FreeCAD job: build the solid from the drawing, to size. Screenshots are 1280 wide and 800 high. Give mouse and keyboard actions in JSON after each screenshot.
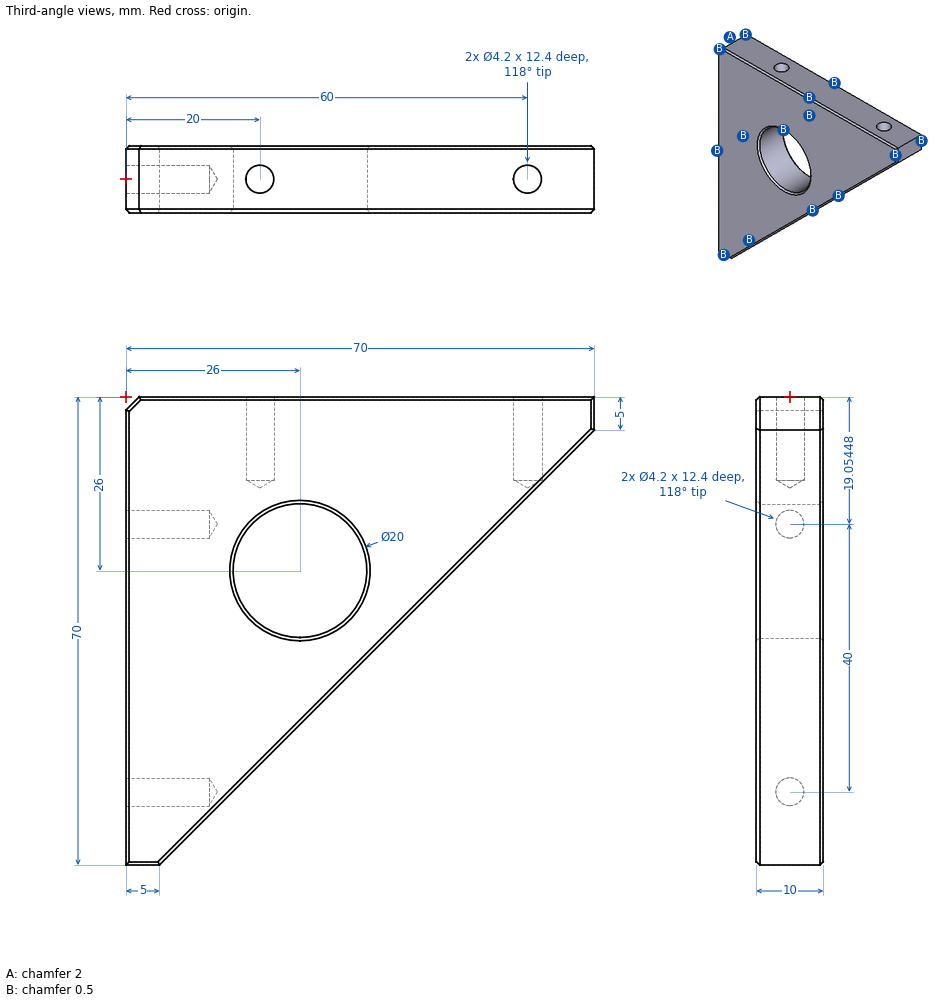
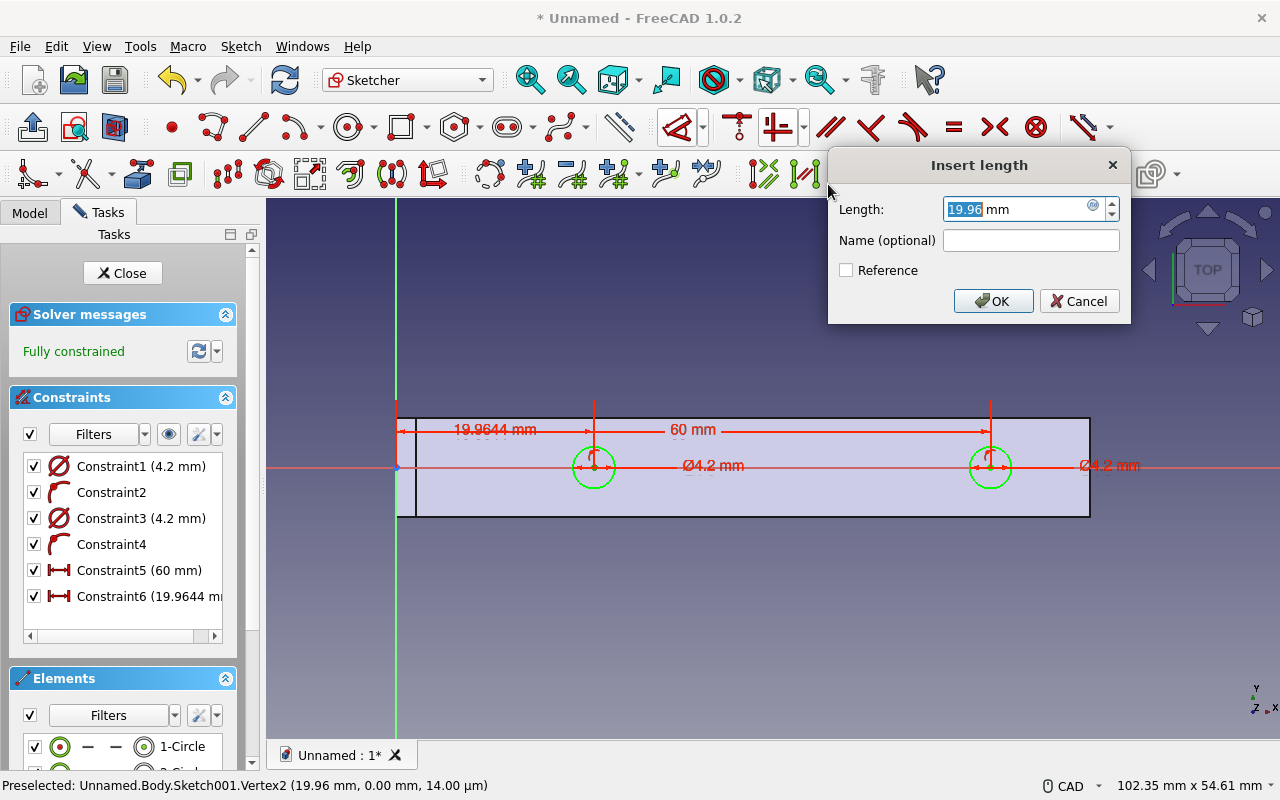
{"action": "type", "text": "20"}
{"action": "key", "text": "Return"}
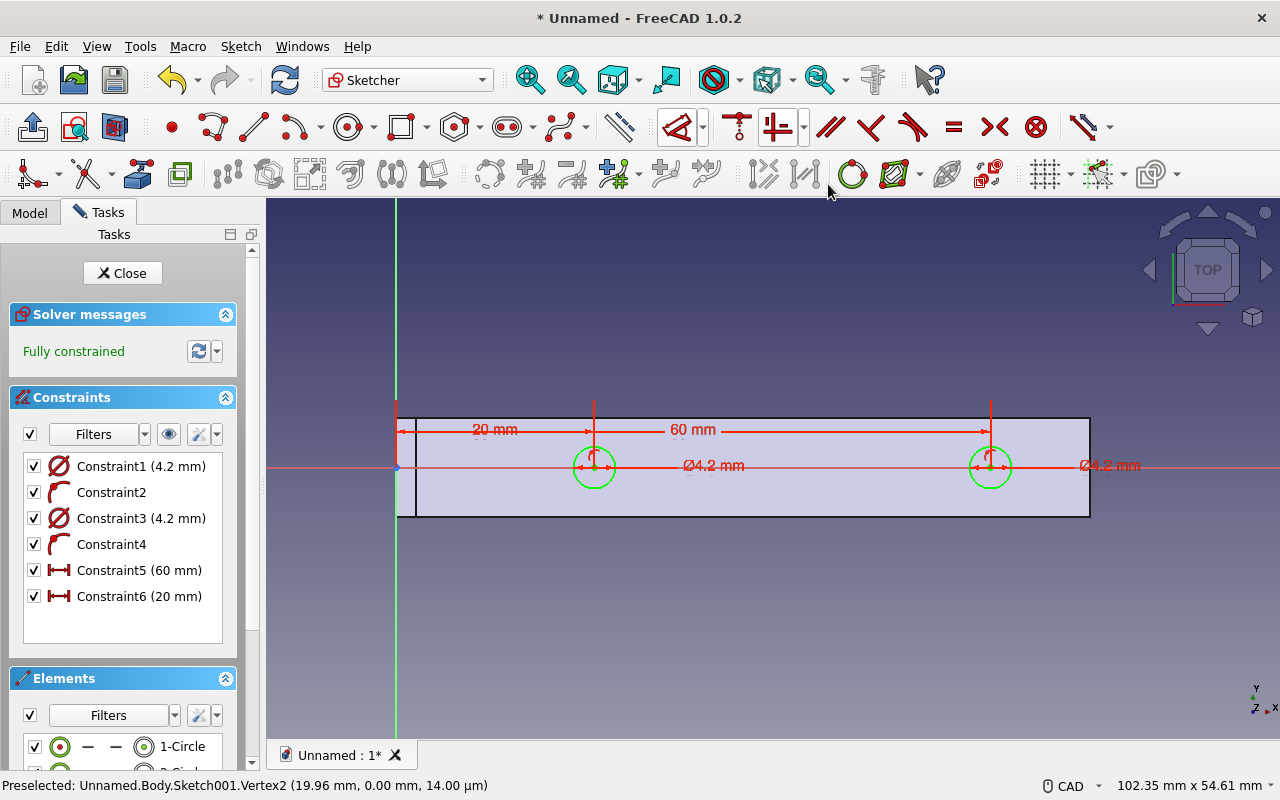
{"action": "left_click", "coordinate": [123, 273]}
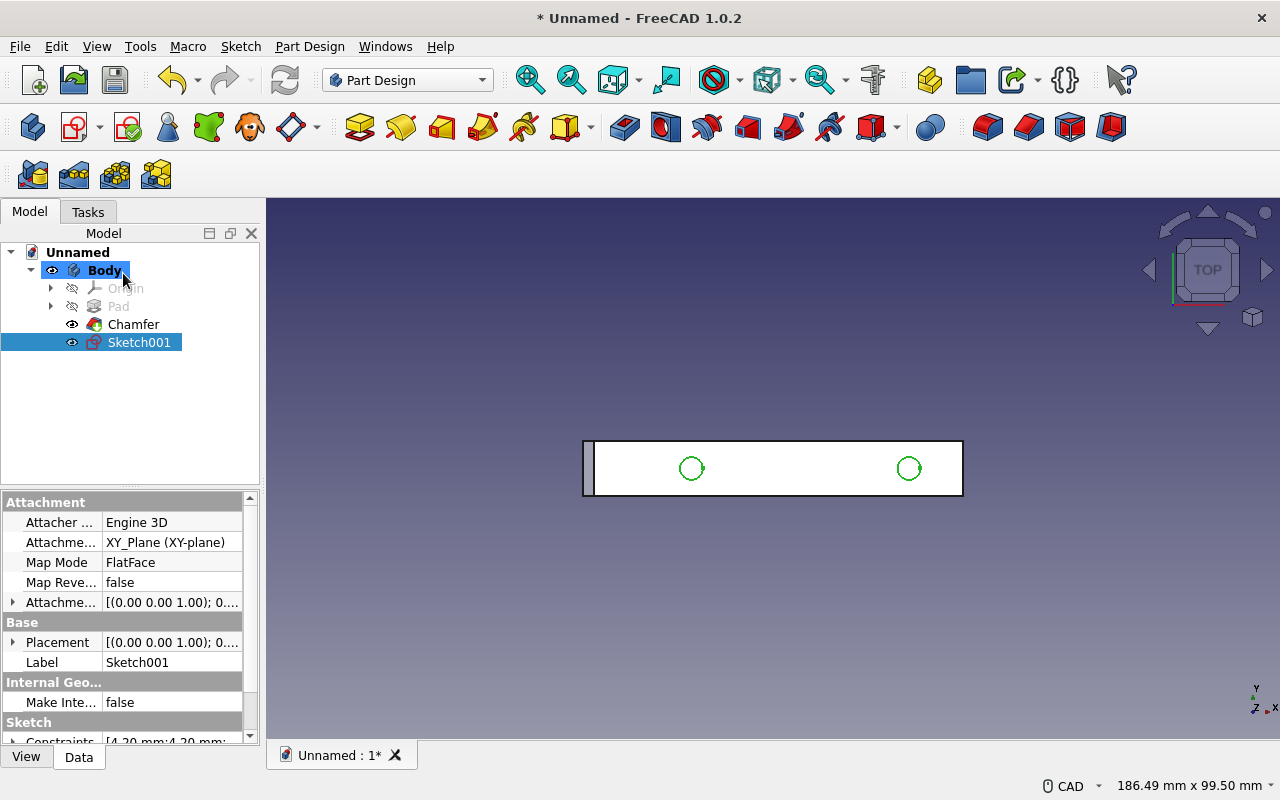
{"action": "left_click", "coordinate": [666, 128]}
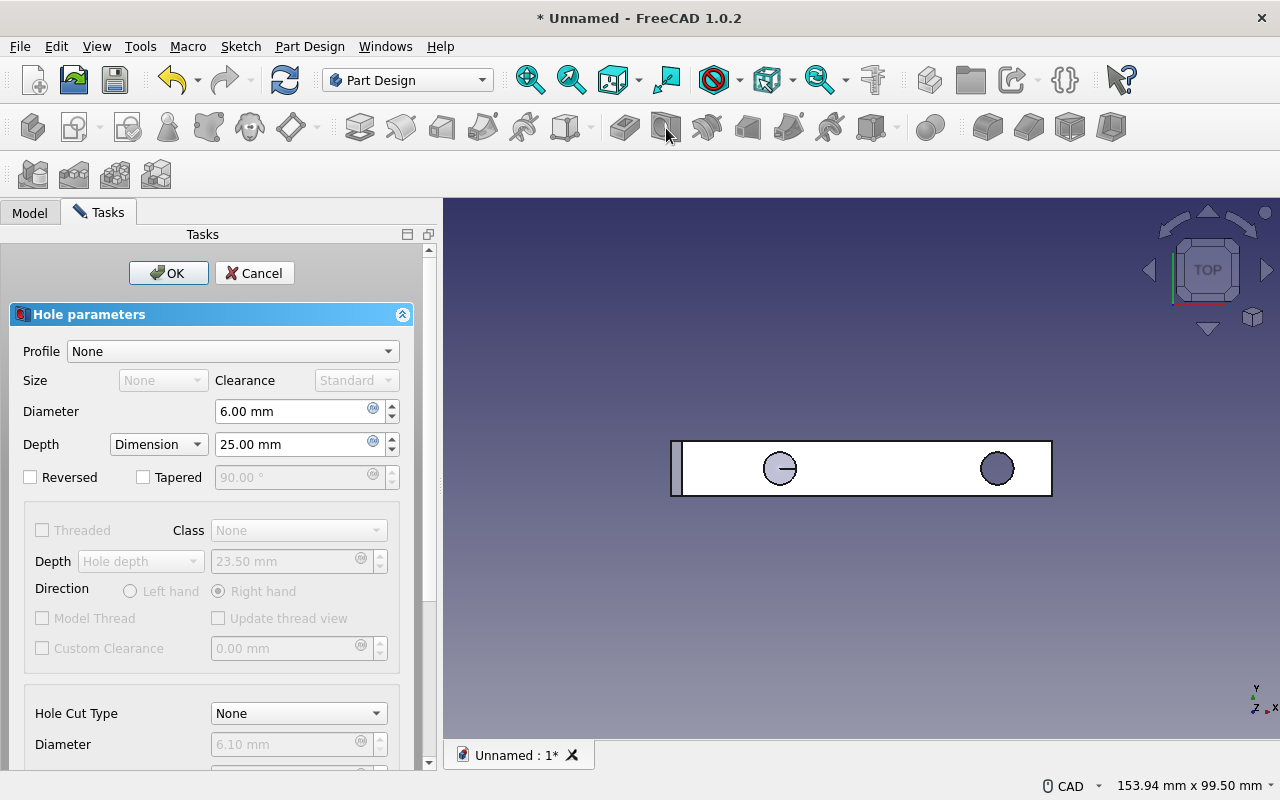
{"action": "triple_click", "coordinate": [300, 412]}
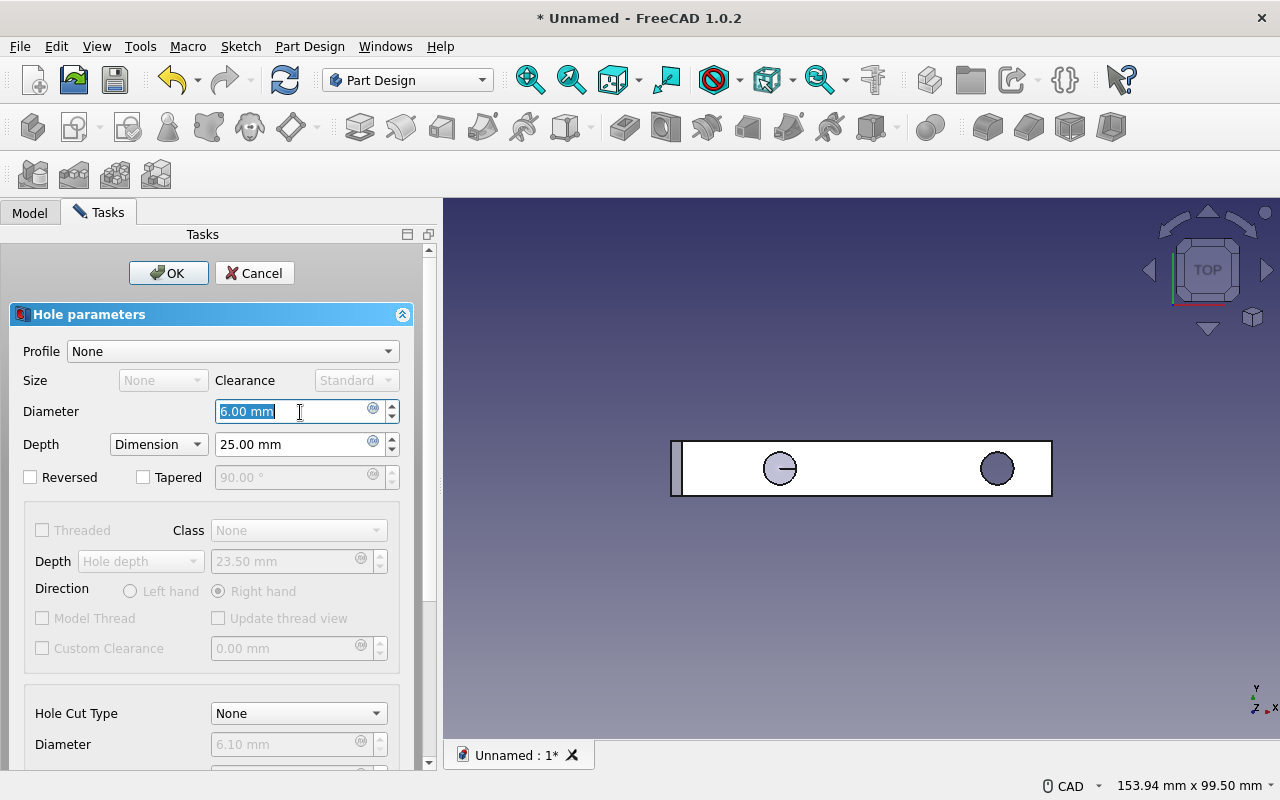
{"action": "type", "text": "4.2"}
{"action": "key", "text": "Tab"}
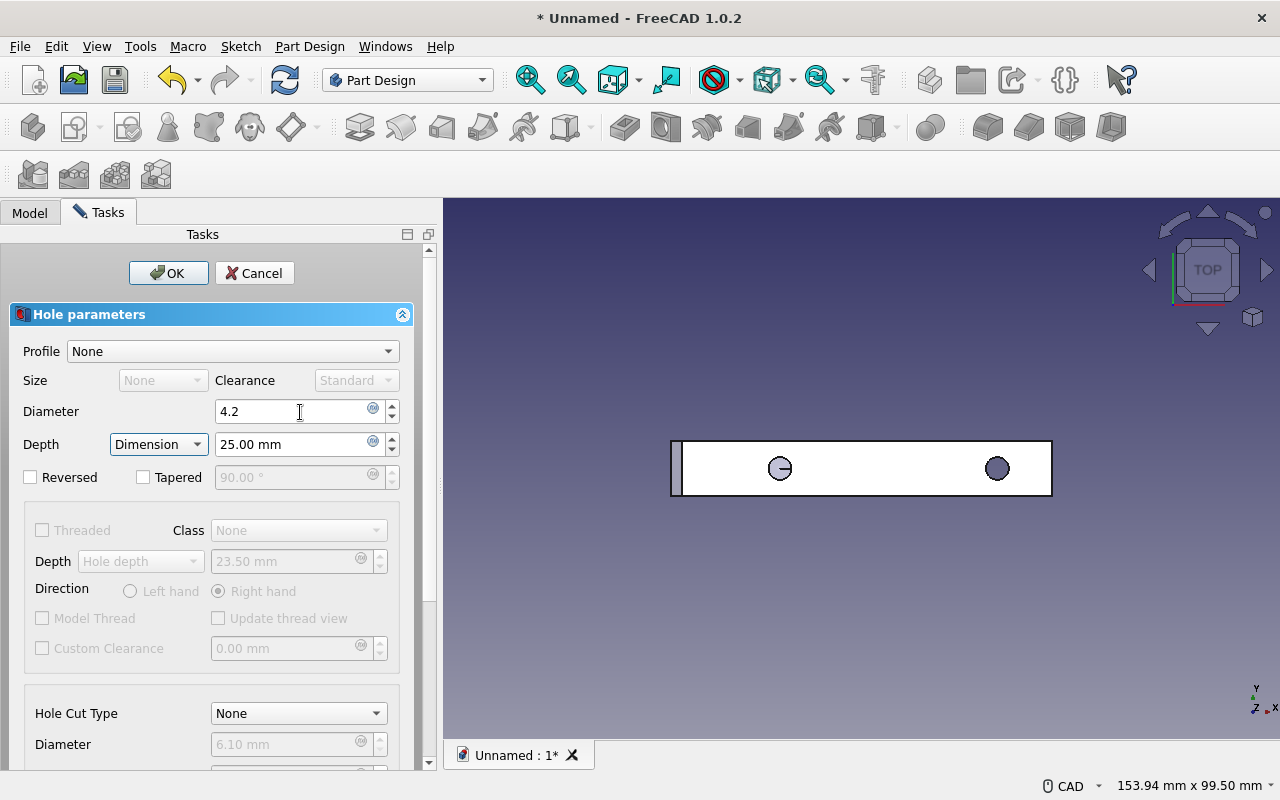
{"action": "triple_click", "coordinate": [300, 444]}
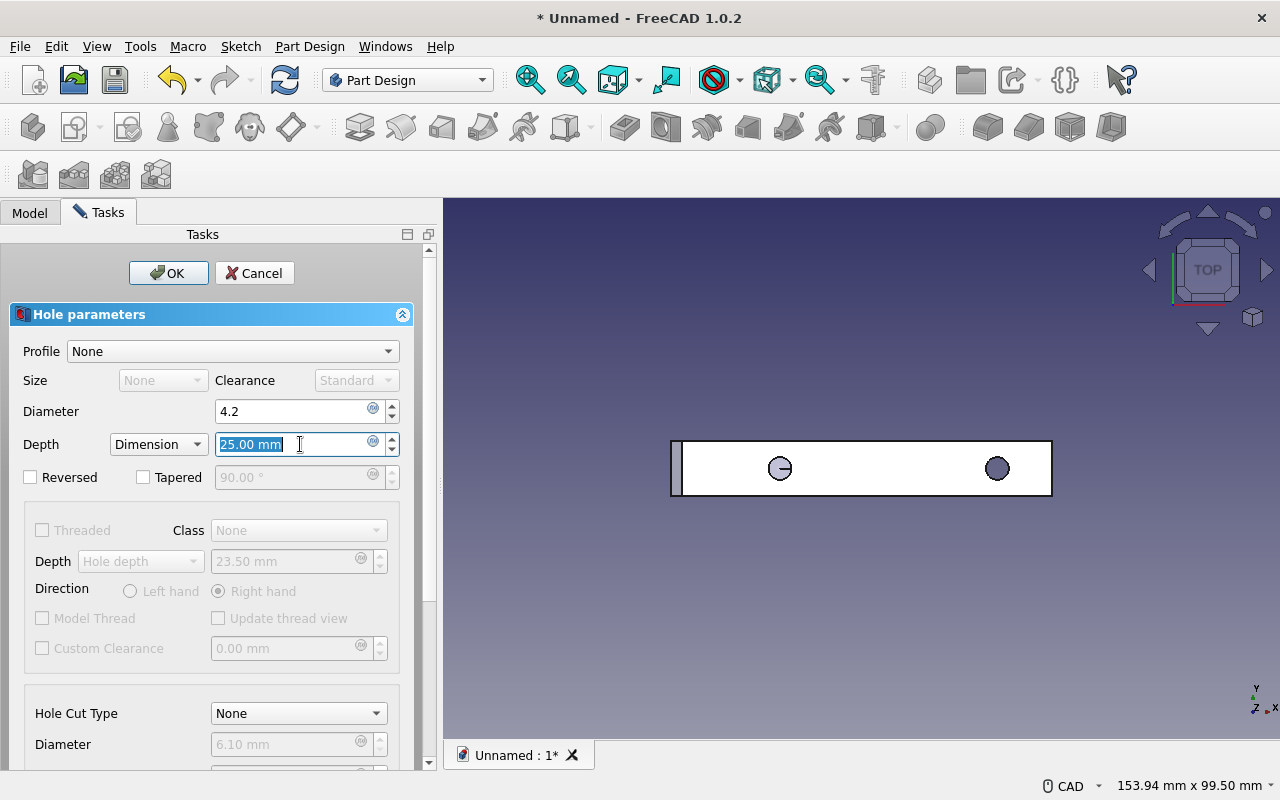
{"action": "type", "text": "12.4"}
{"action": "key", "text": "Tab"}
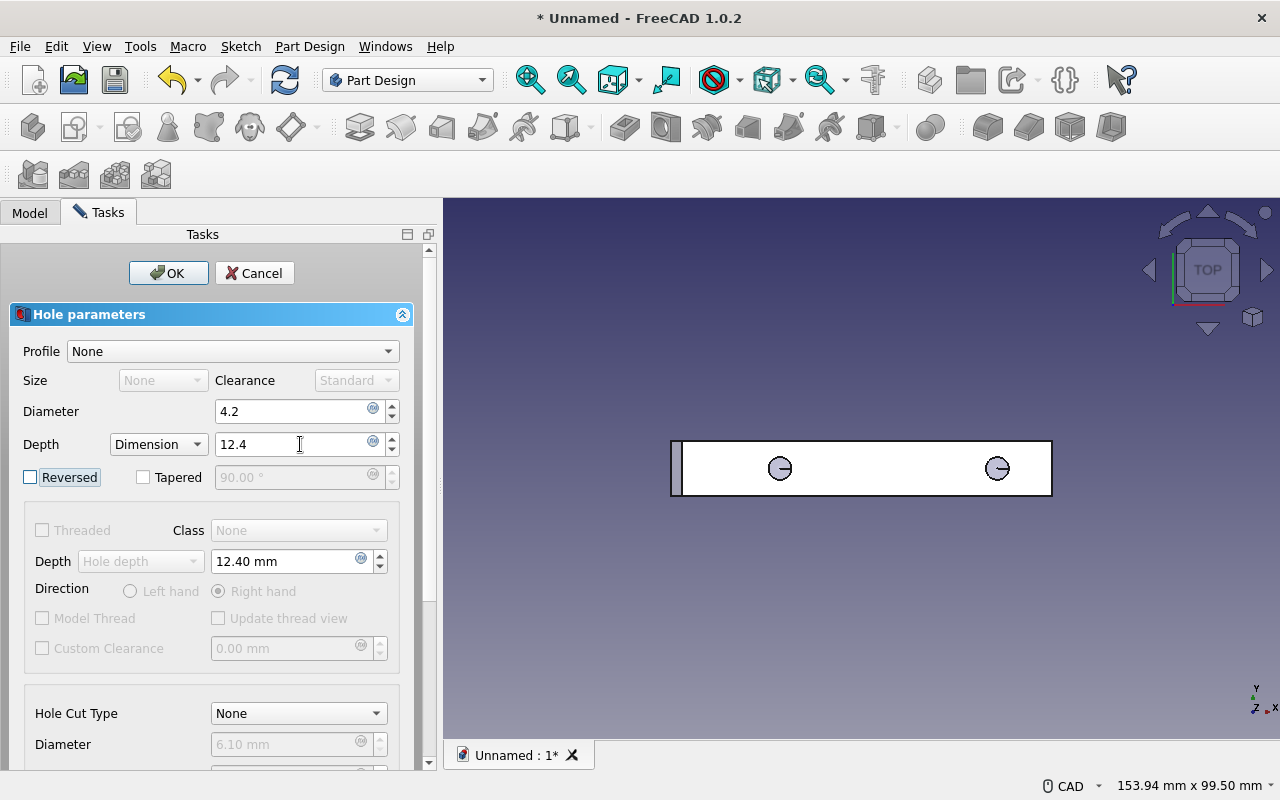
{"action": "left_click", "coordinate": [169, 273]}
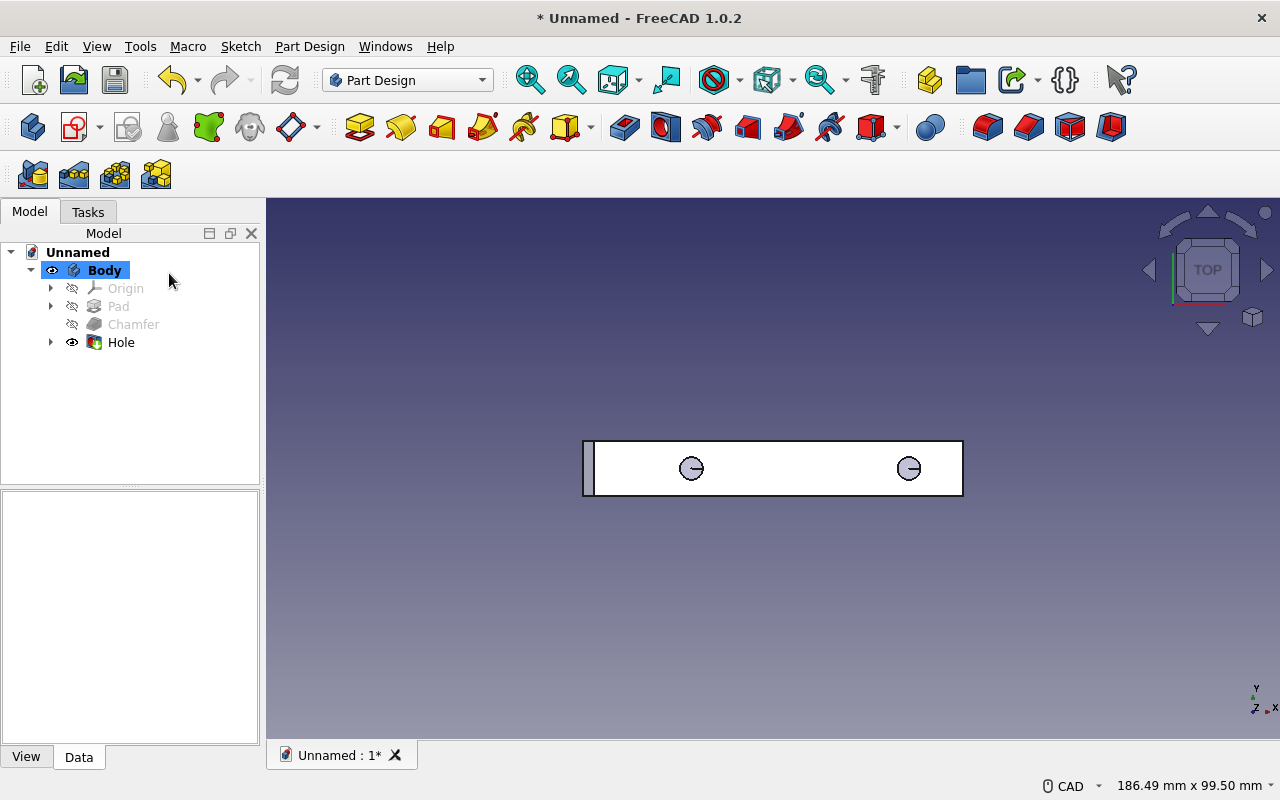
{"action": "left_click", "coordinate": [531, 80]}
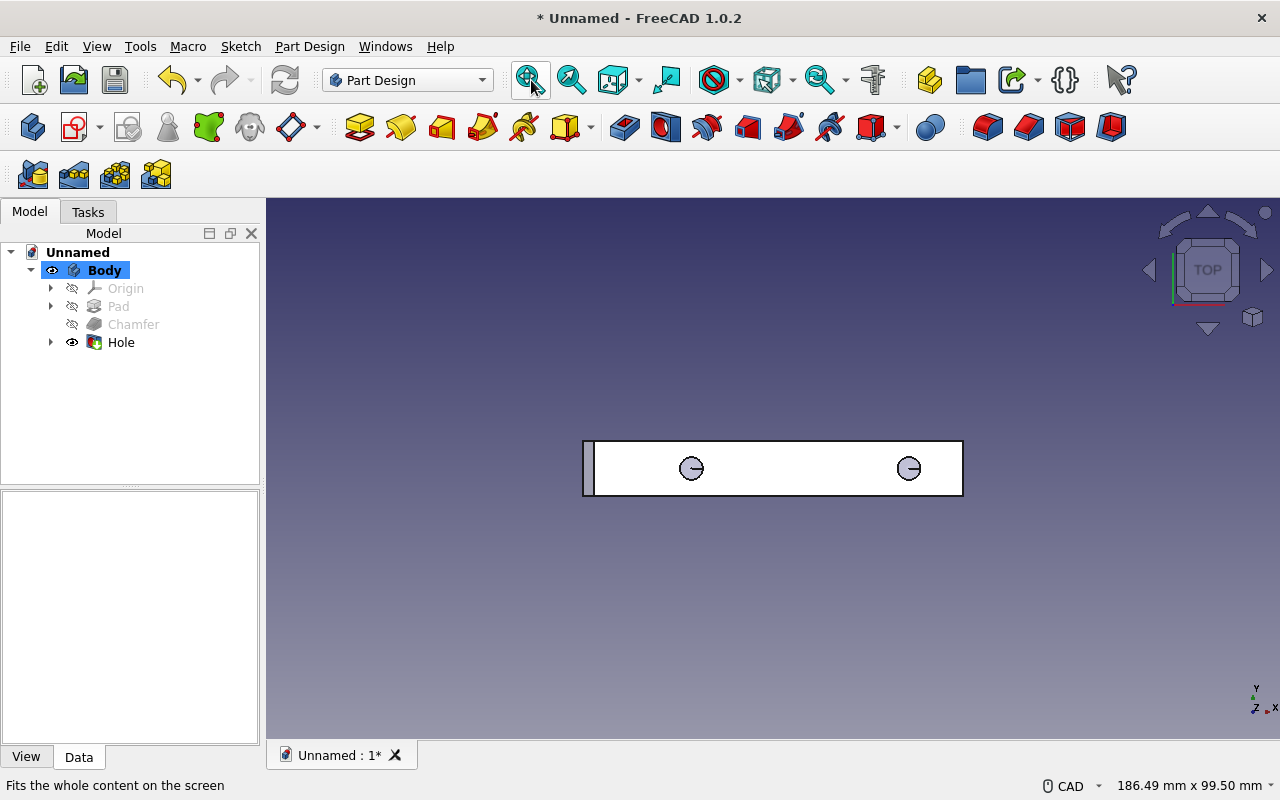
{"action": "key", "text": "6"}